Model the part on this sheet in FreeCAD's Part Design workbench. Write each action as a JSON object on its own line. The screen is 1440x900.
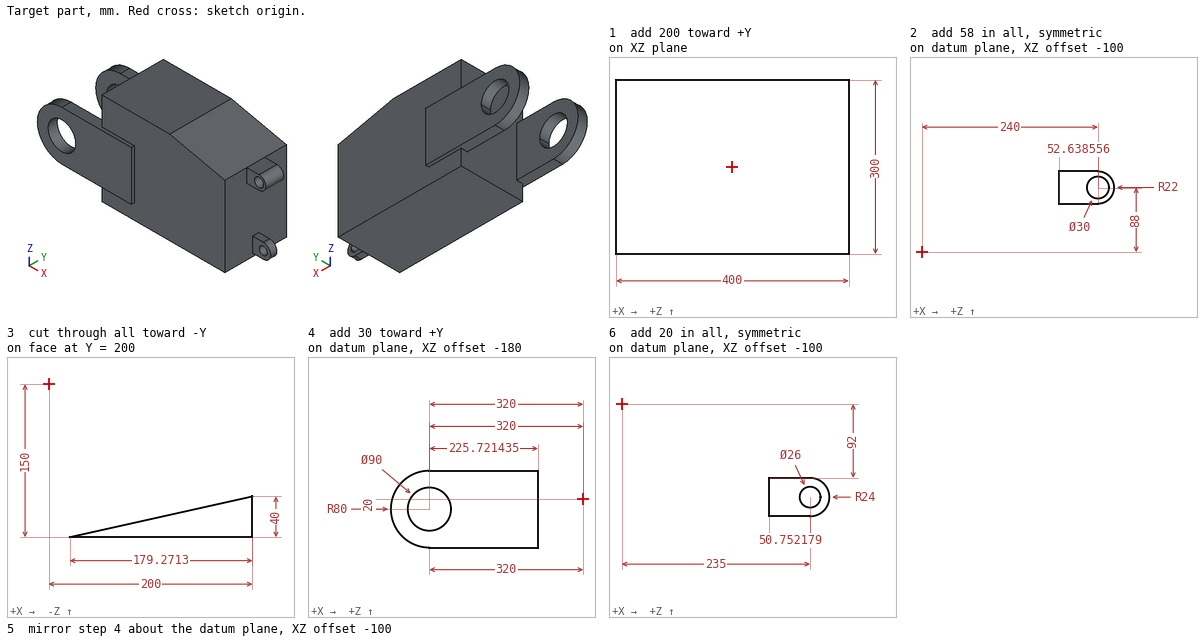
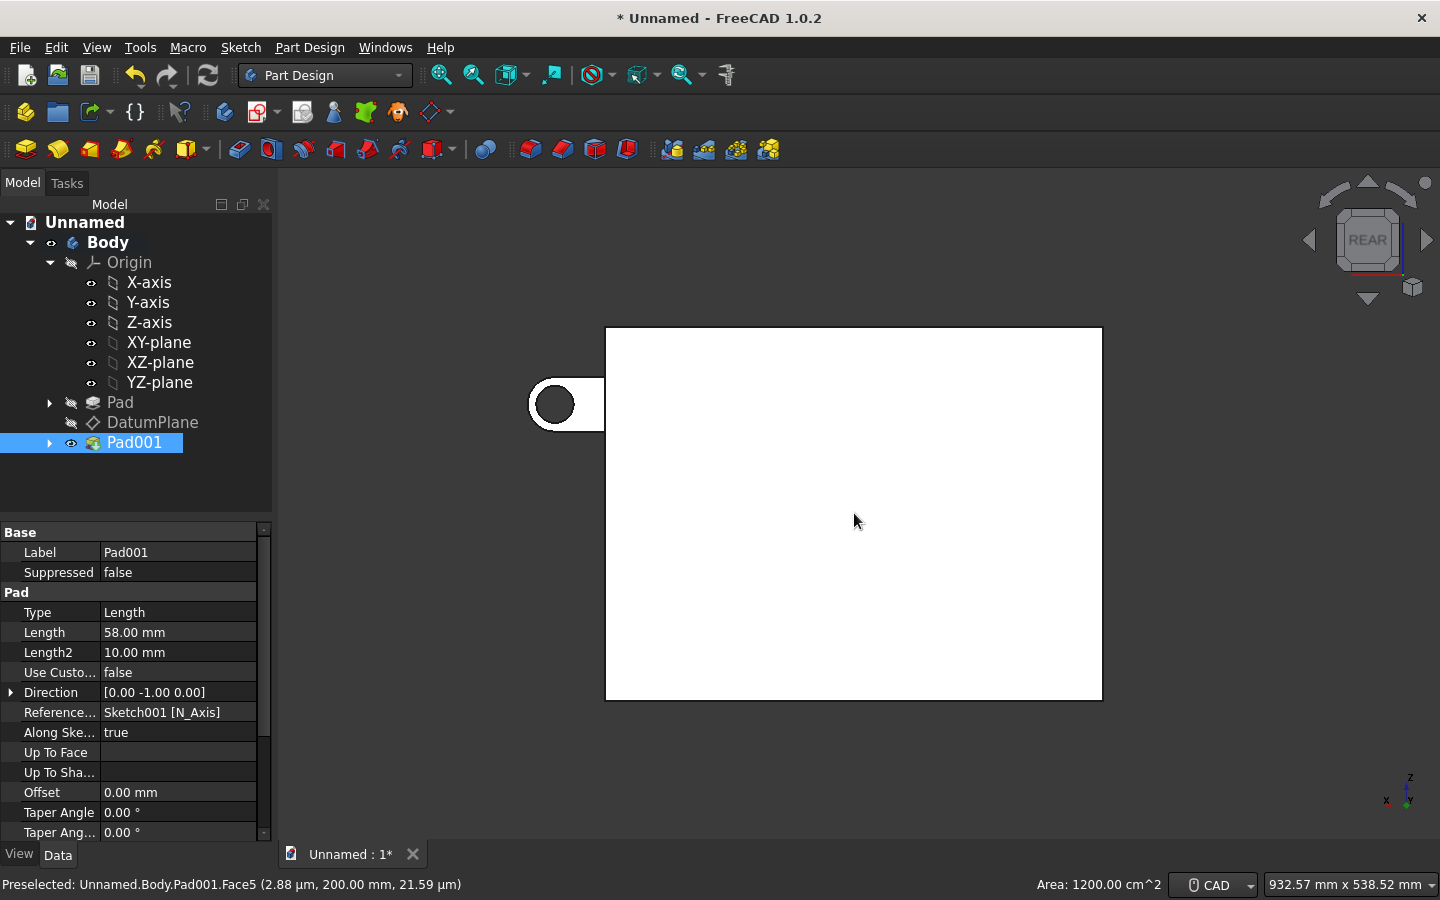
{"action": "left_click", "coordinate": [258, 112]}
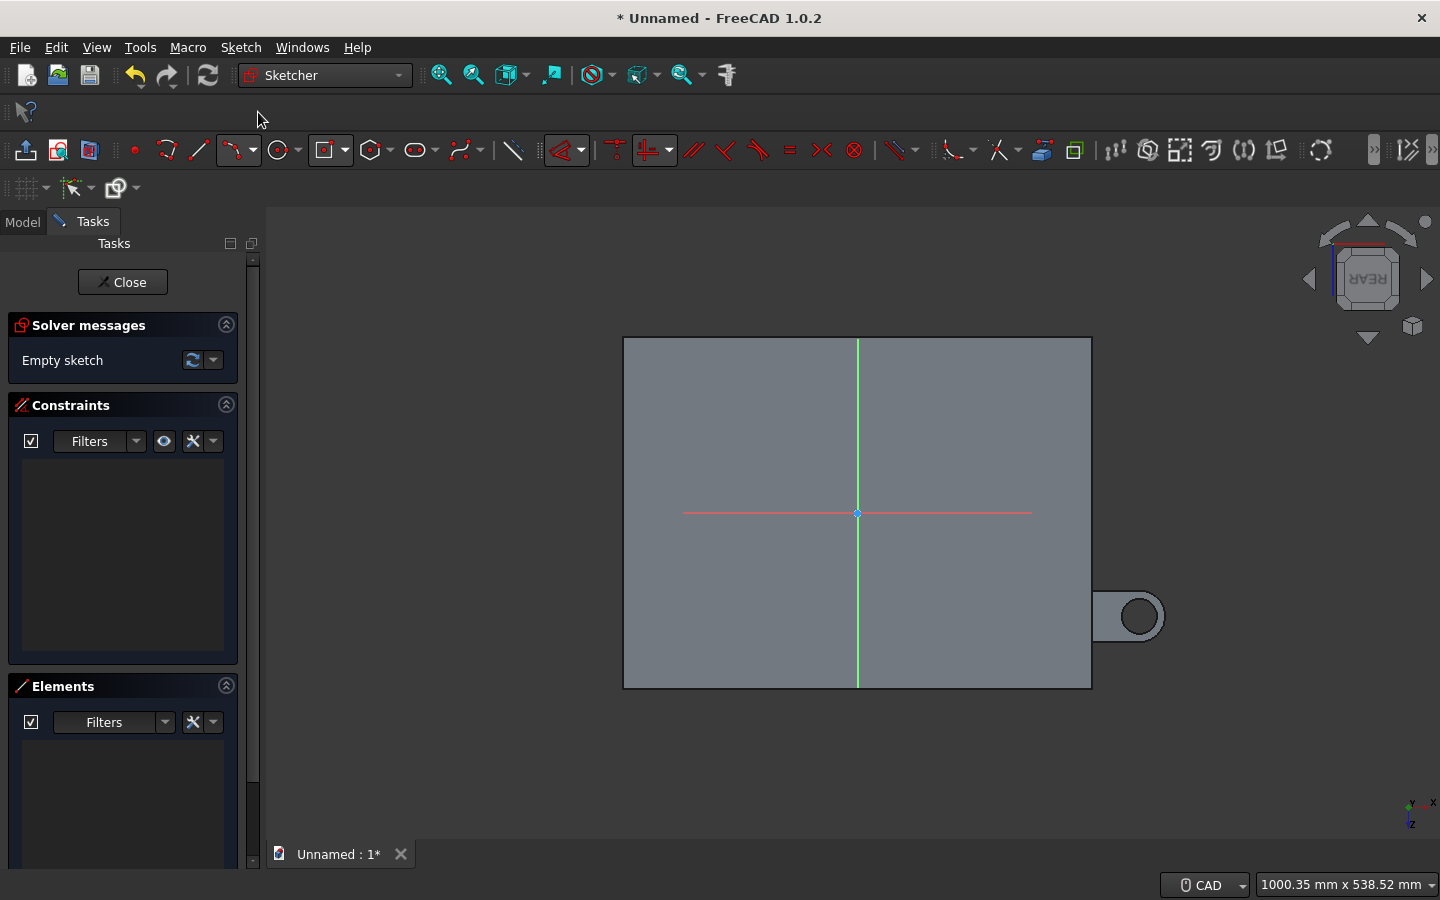
{"action": "scroll", "coordinate": [1131, 665], "scroll_direction": "up", "scroll_amount": 4}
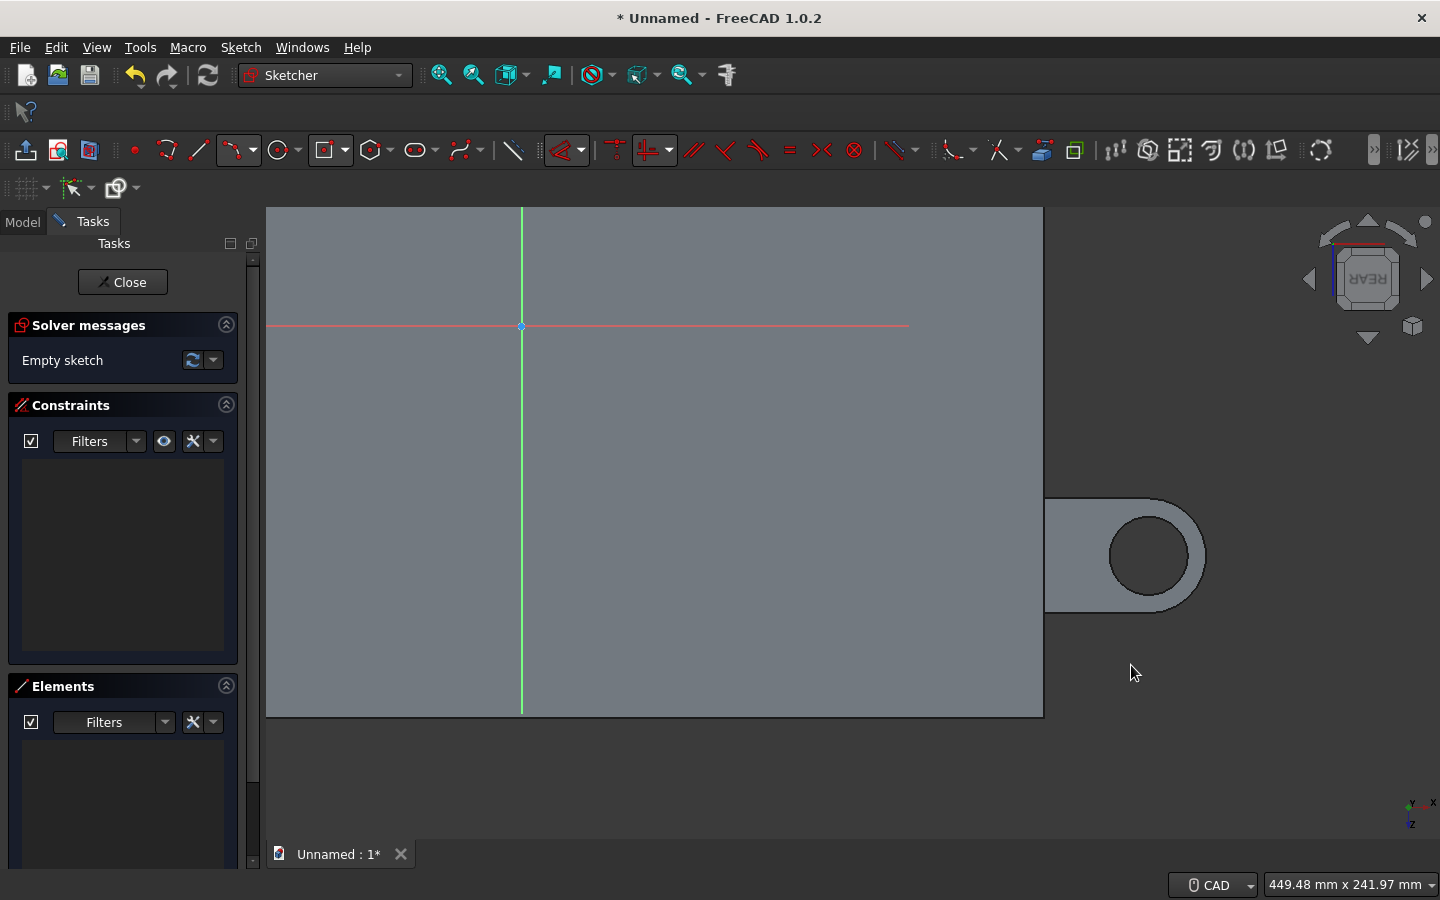
{"action": "left_click", "coordinate": [168, 150]}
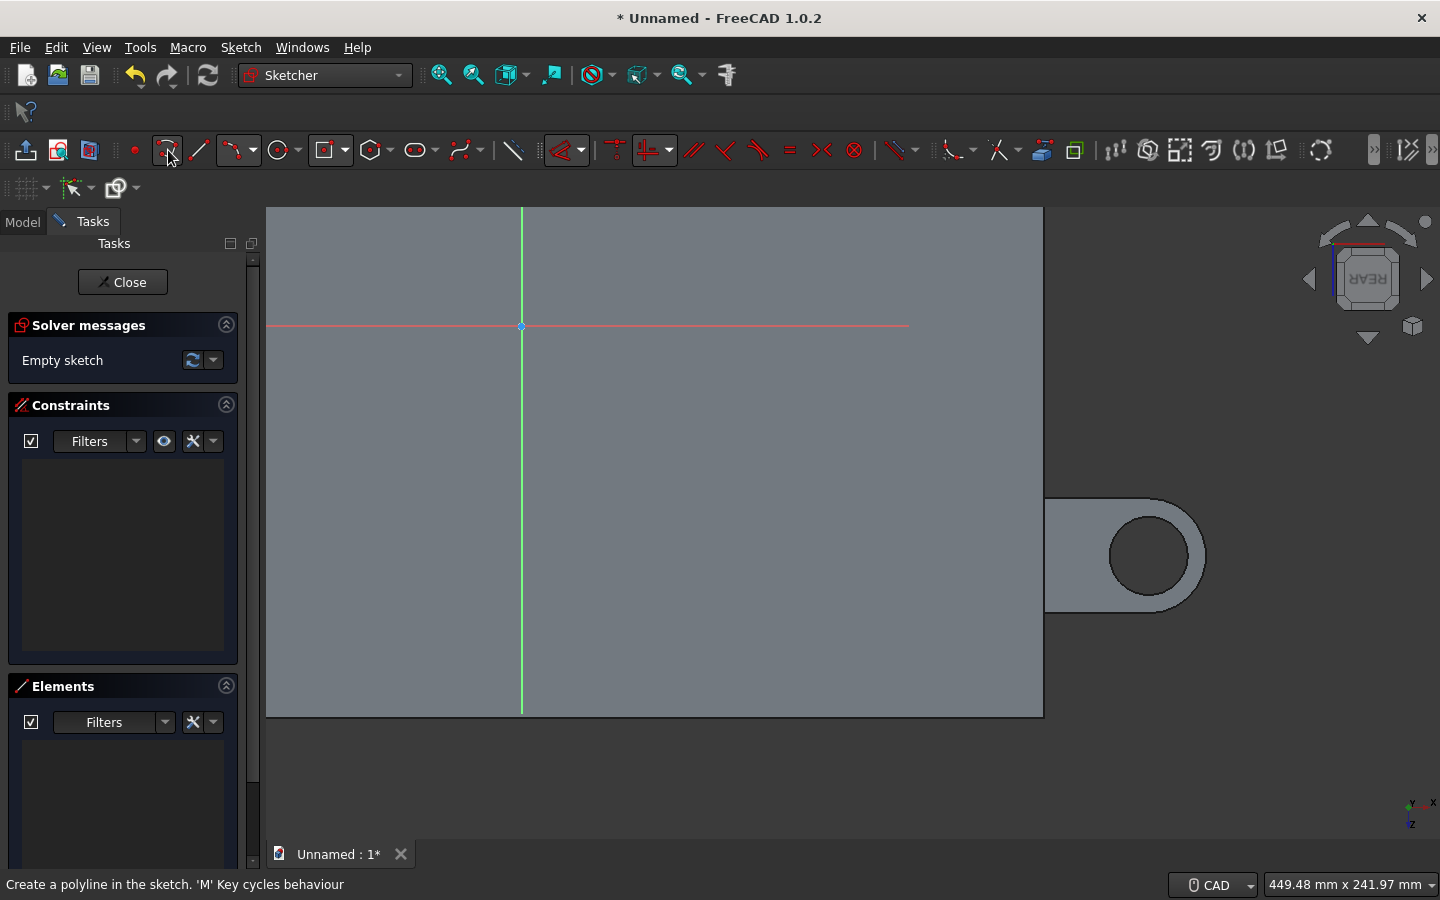
{"action": "left_click", "coordinate": [576, 718]}
{"action": "left_click", "coordinate": [1044, 718]}
{"action": "left_click", "coordinate": [1044, 613]}
{"action": "left_click", "coordinate": [576, 719]}
{"action": "key", "text": "Escape"}
{"action": "key", "text": "Escape"}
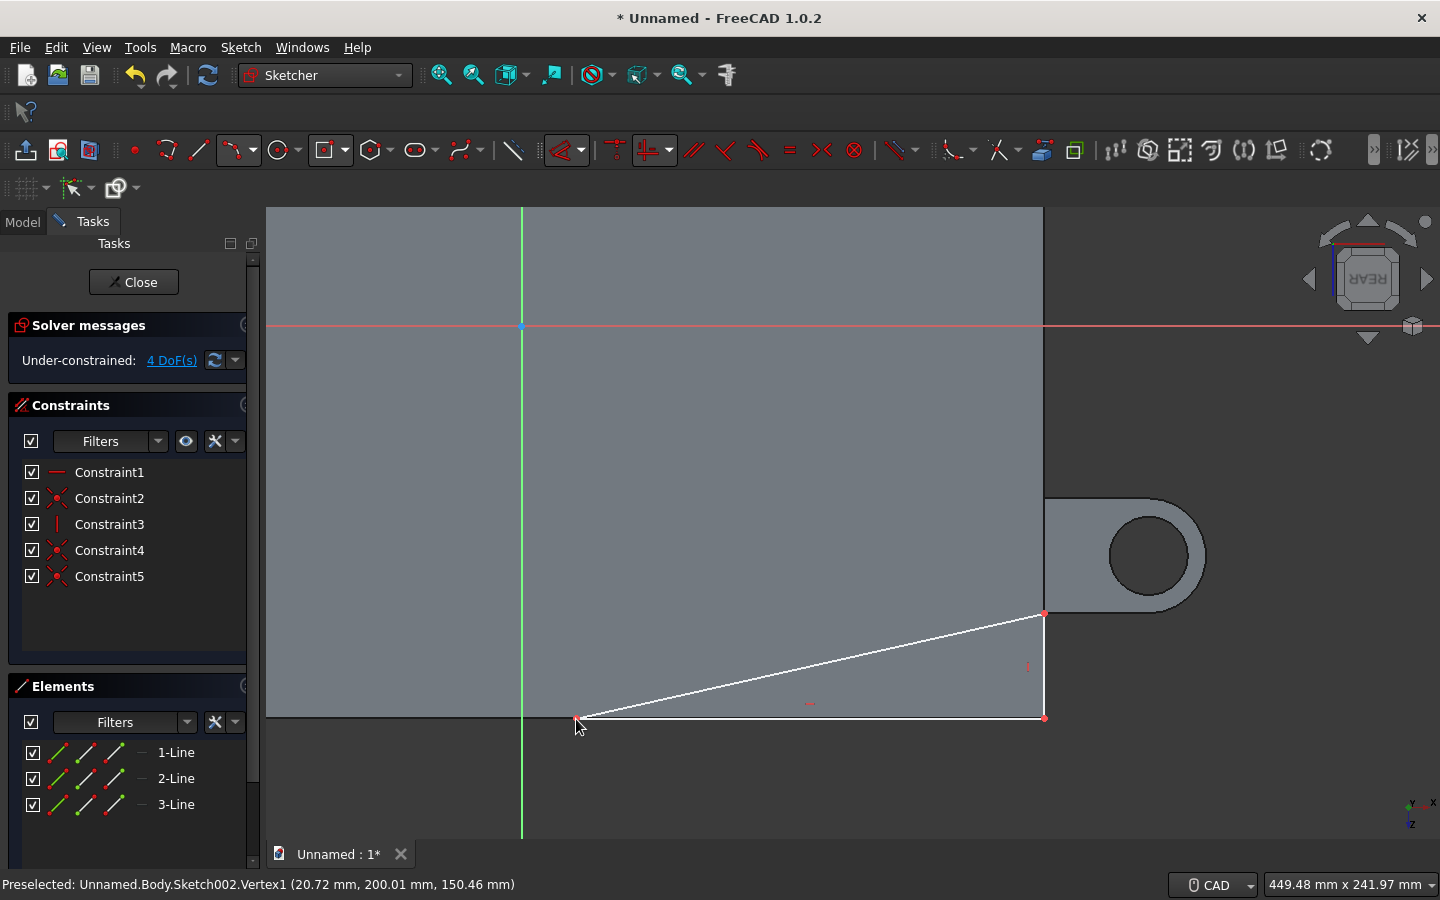
{"action": "left_click", "coordinate": [1044, 688]}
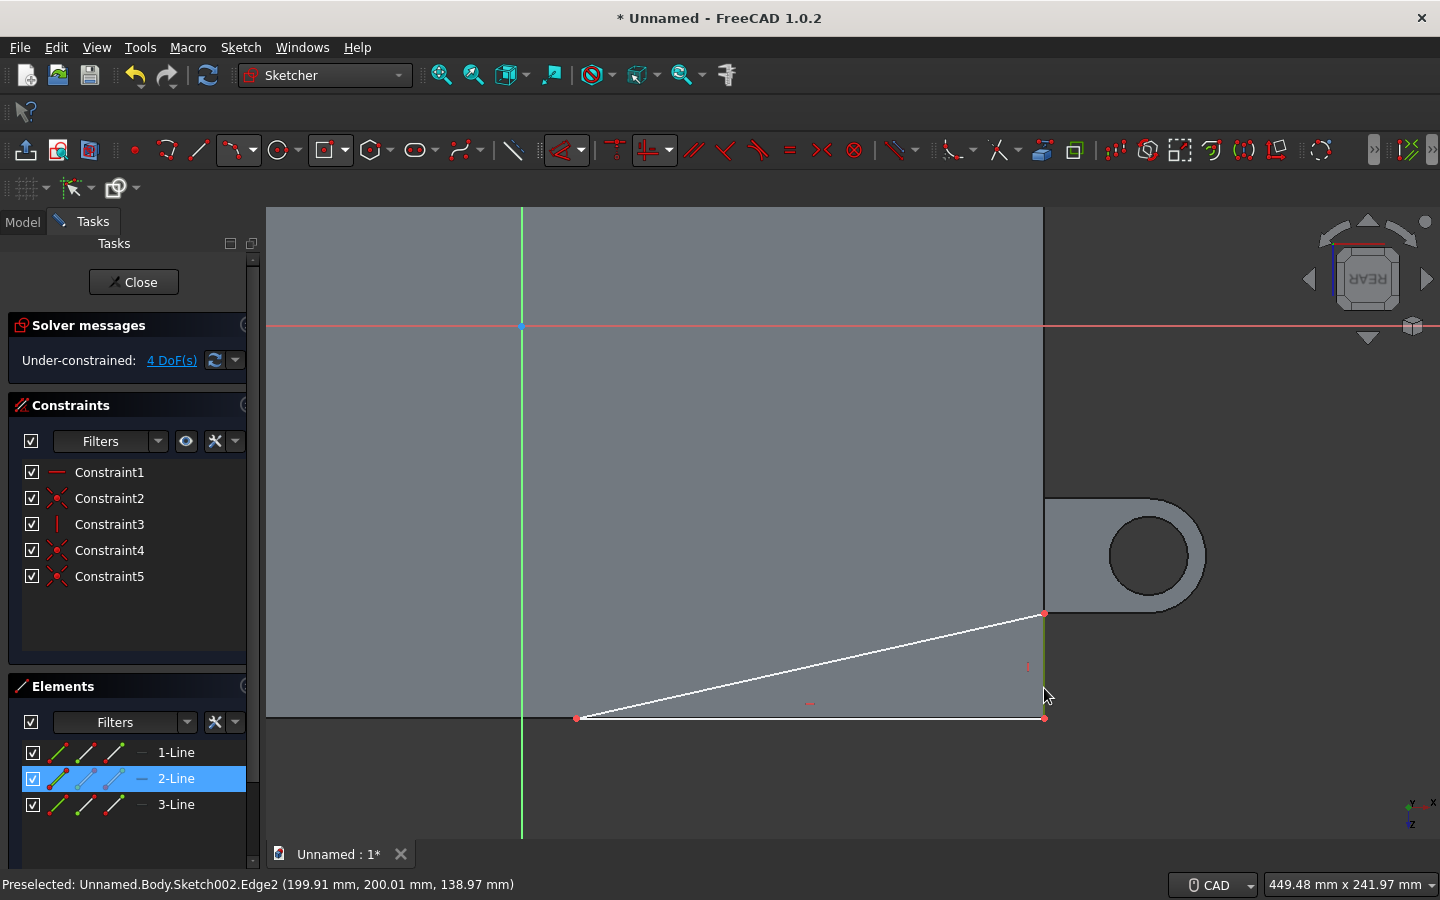
{"action": "left_click", "coordinate": [584, 150]}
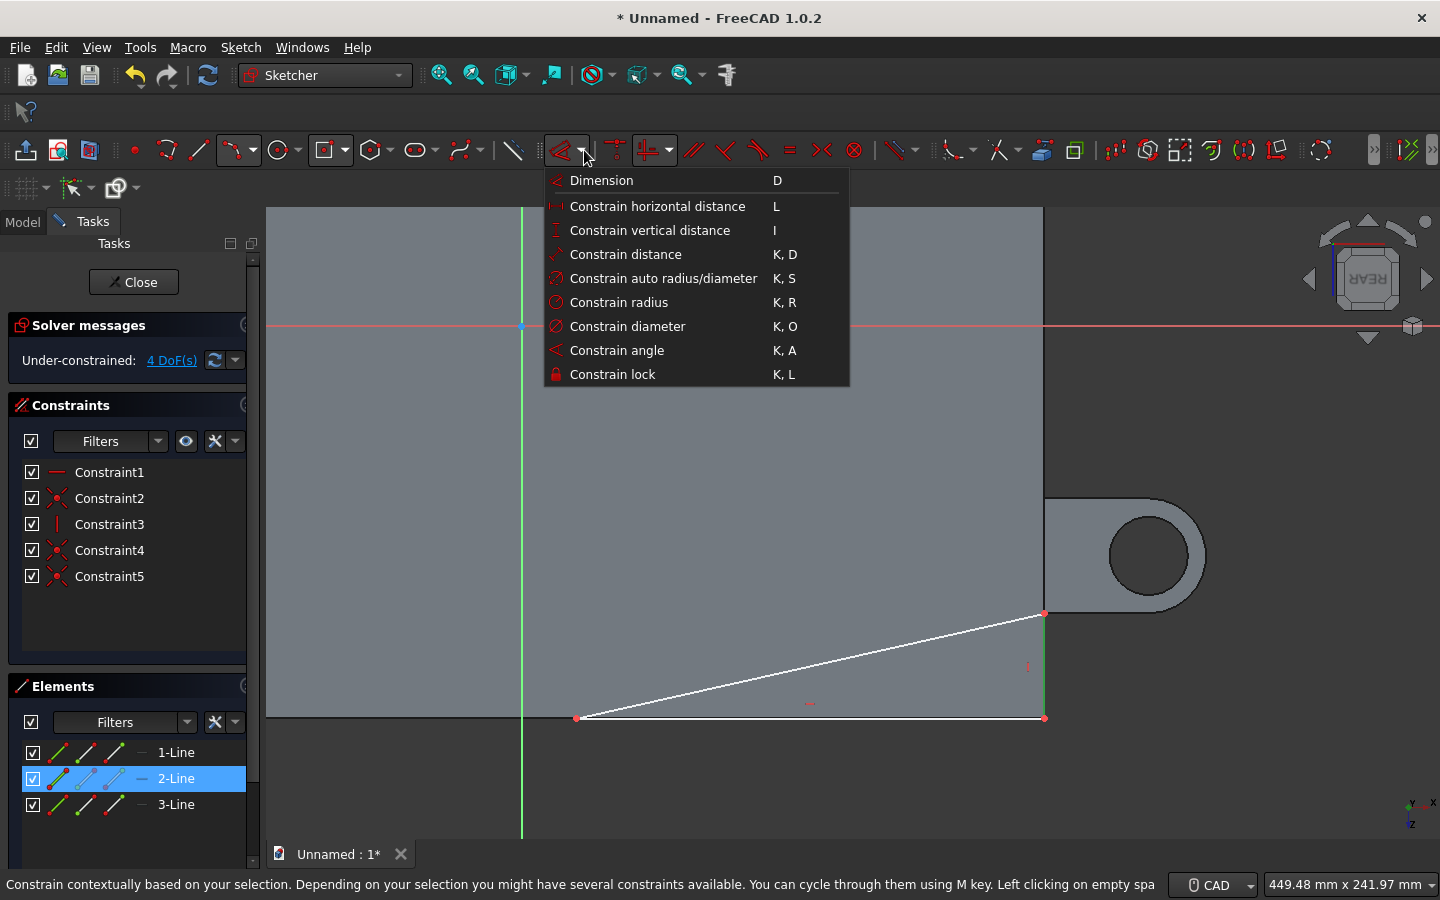
{"action": "left_click", "coordinate": [697, 230]}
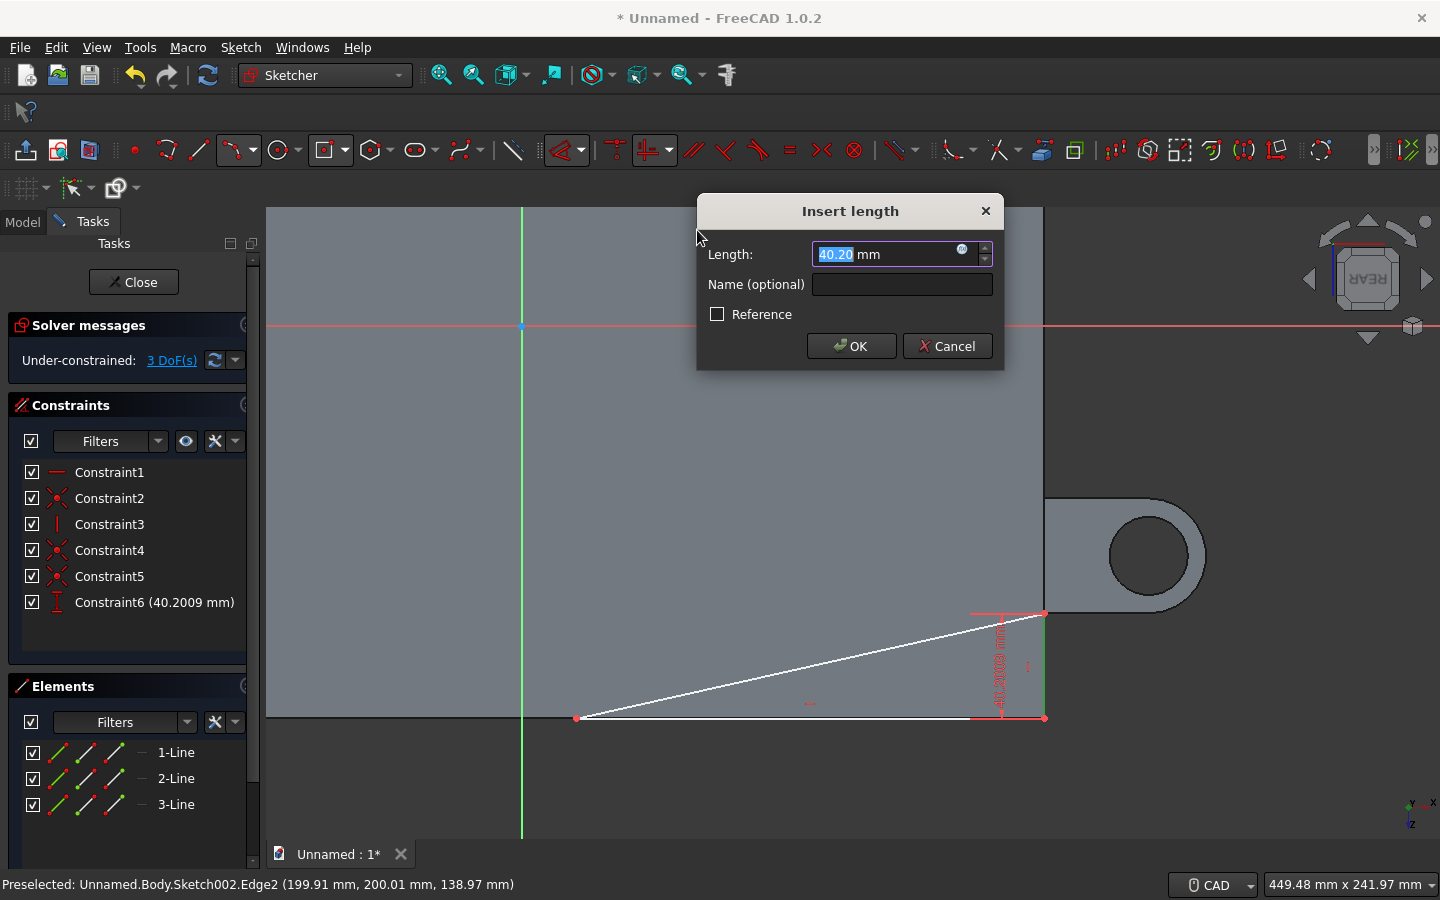
{"action": "type", "text": "40"}
{"action": "key", "text": "Return"}